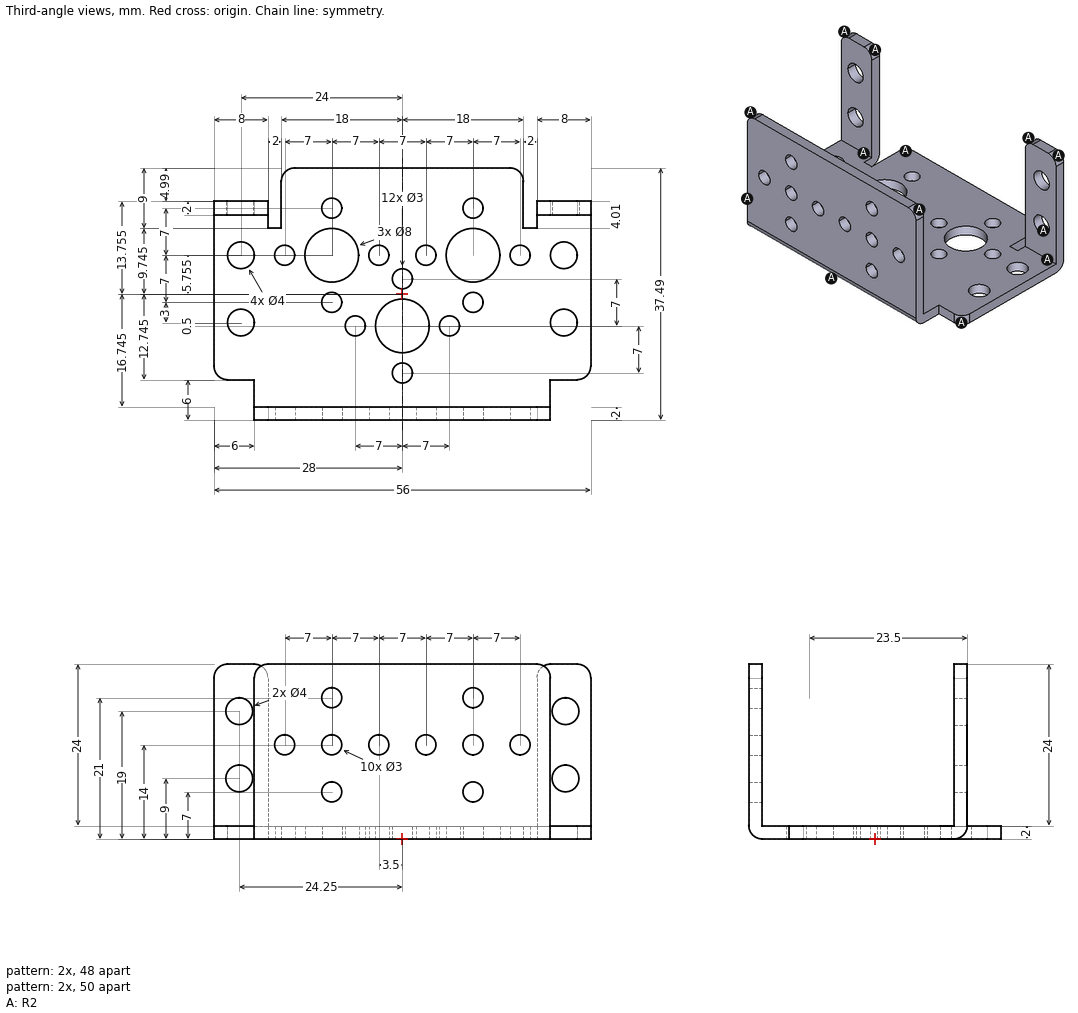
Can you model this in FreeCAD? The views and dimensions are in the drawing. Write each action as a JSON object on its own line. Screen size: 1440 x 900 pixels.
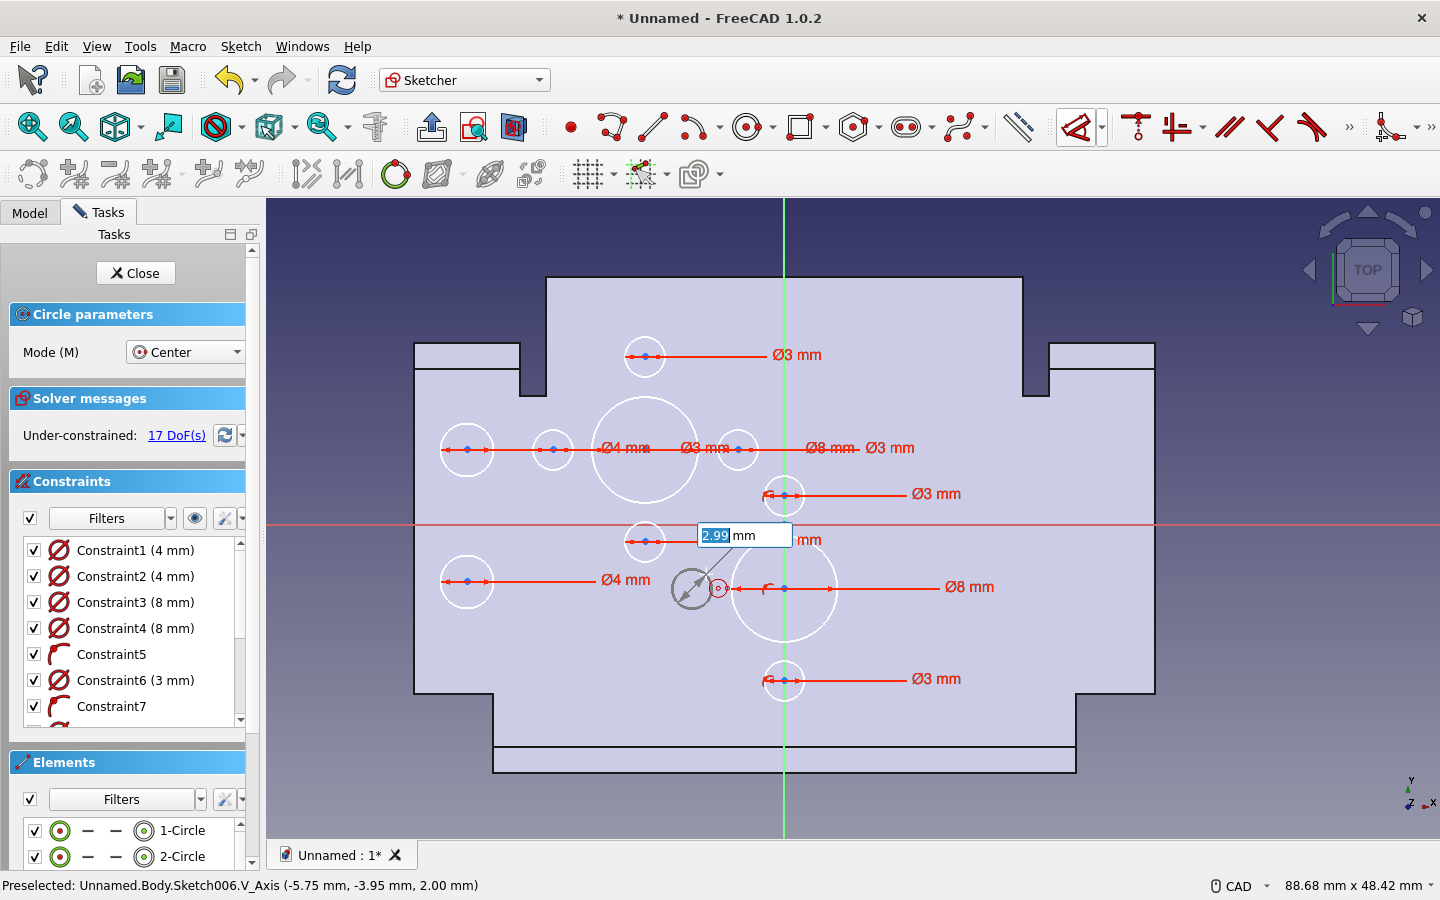
{"action": "type", "text": "3"}
{"action": "key", "text": "Return"}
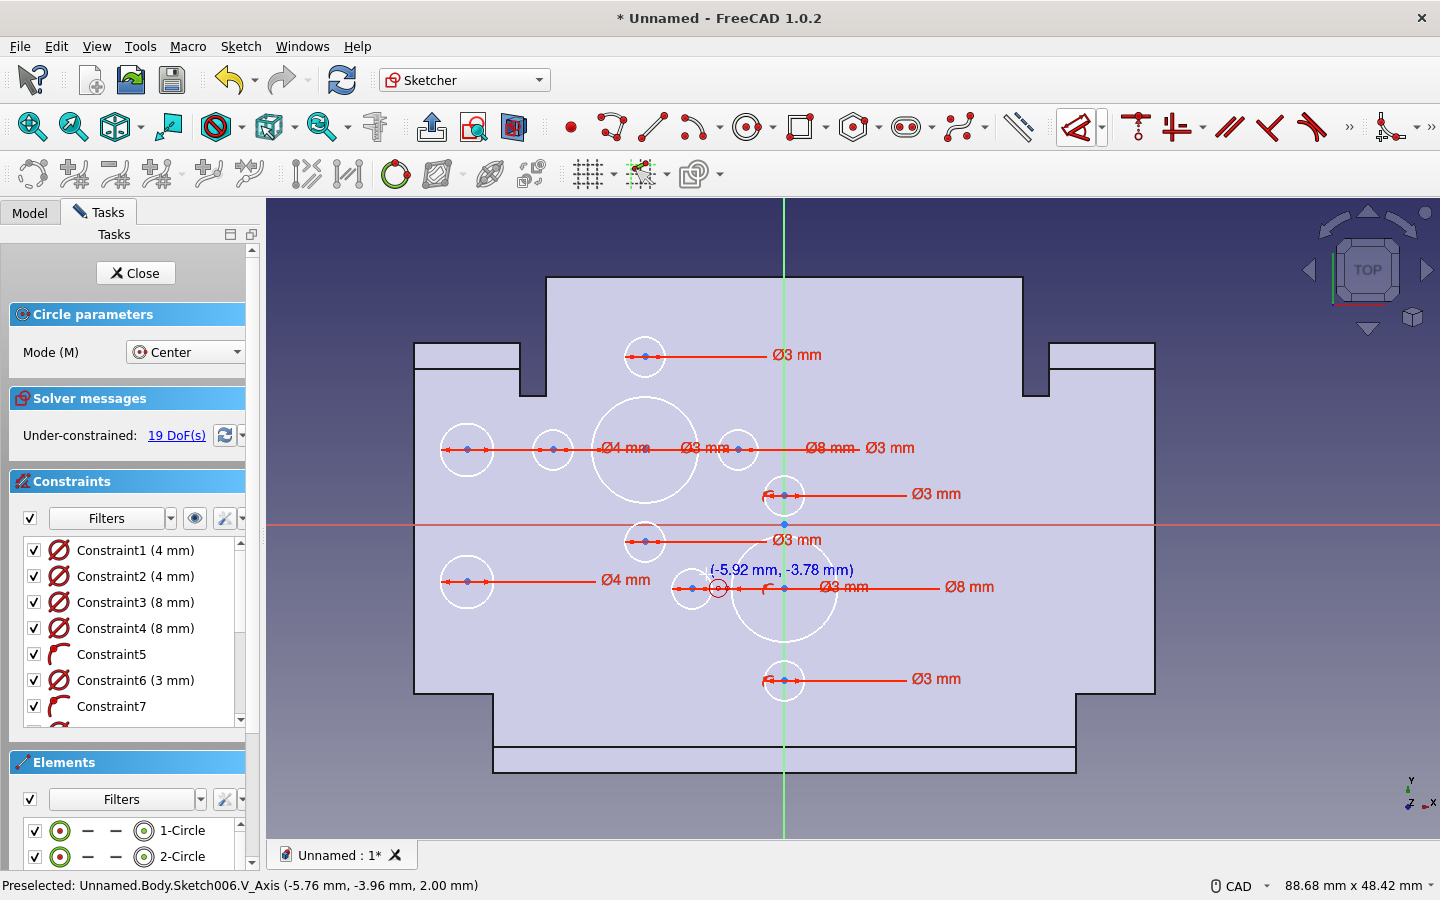
{"action": "left_click", "coordinate": [877, 588]}
{"action": "mouse_move", "coordinate": [891, 574]}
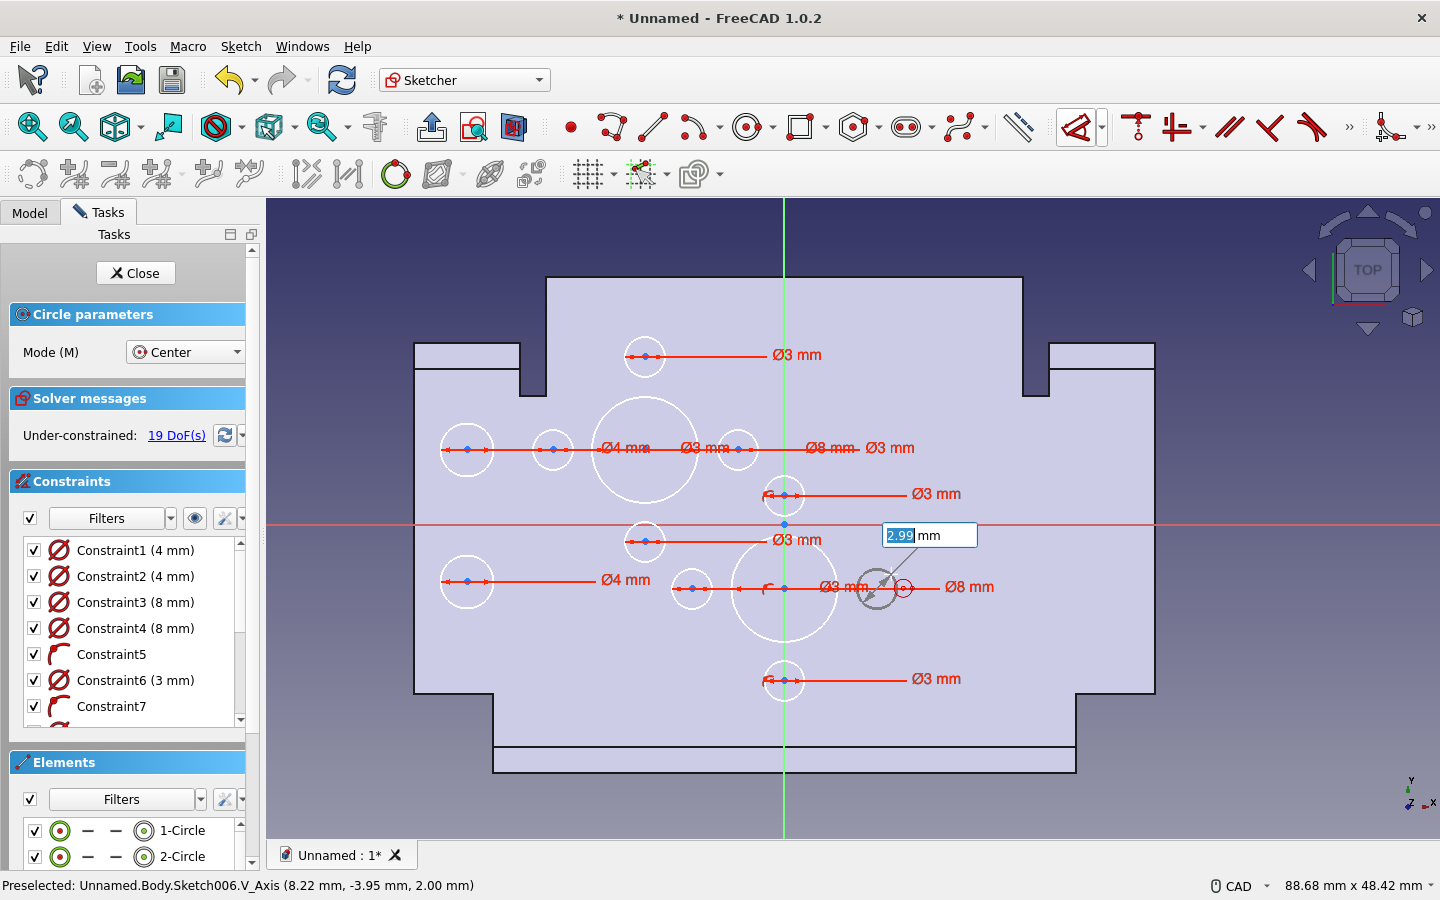
{"action": "type", "text": "3"}
{"action": "key", "text": "Return"}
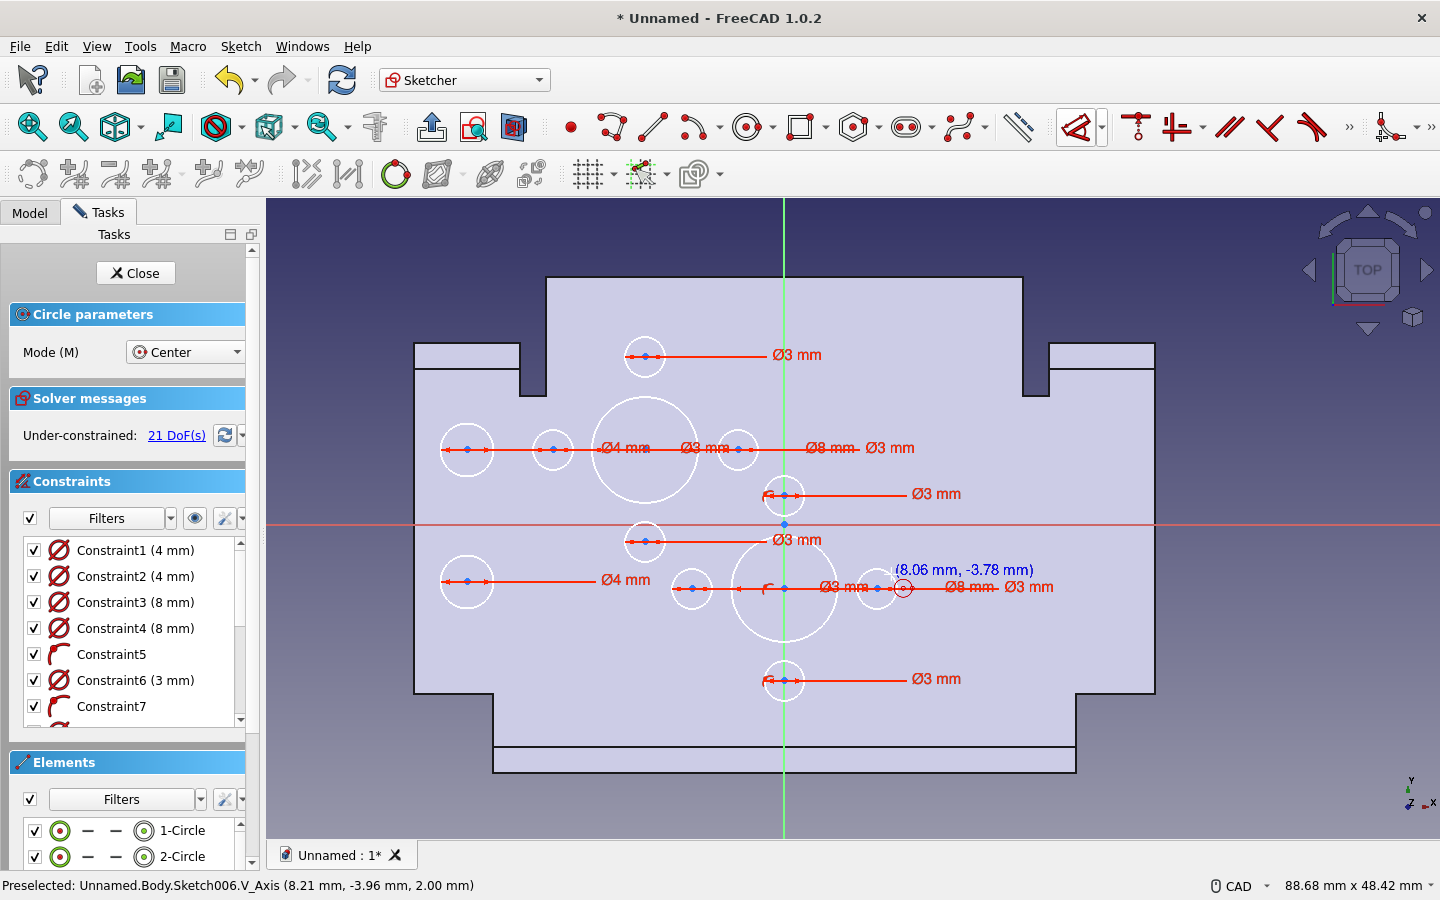
{"action": "left_click", "coordinate": [923, 356]}
{"action": "mouse_move", "coordinate": [937, 342]}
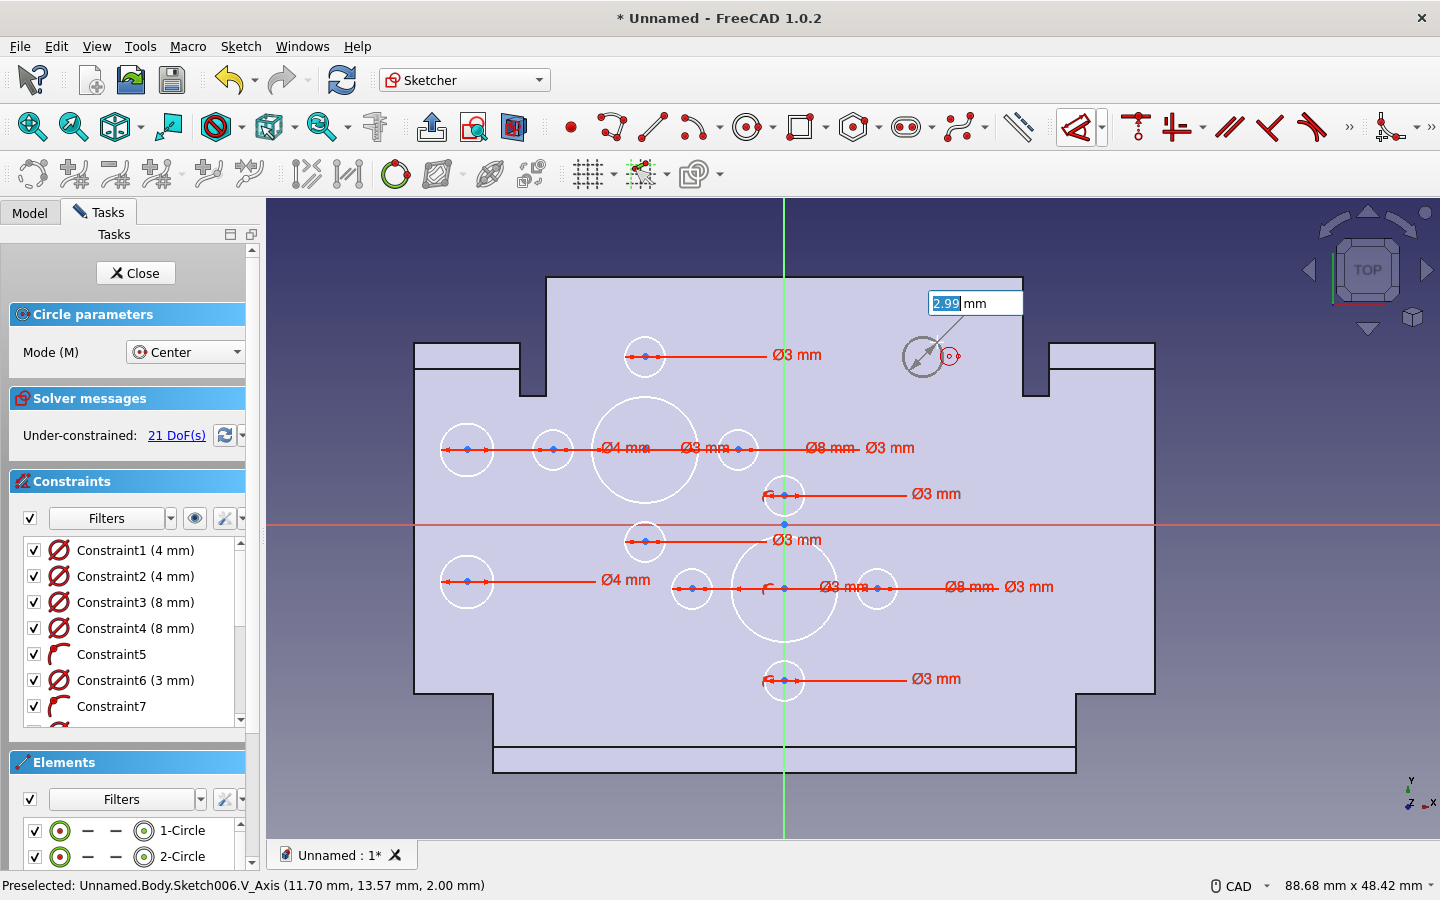
{"action": "type", "text": "3"}
{"action": "key", "text": "Return"}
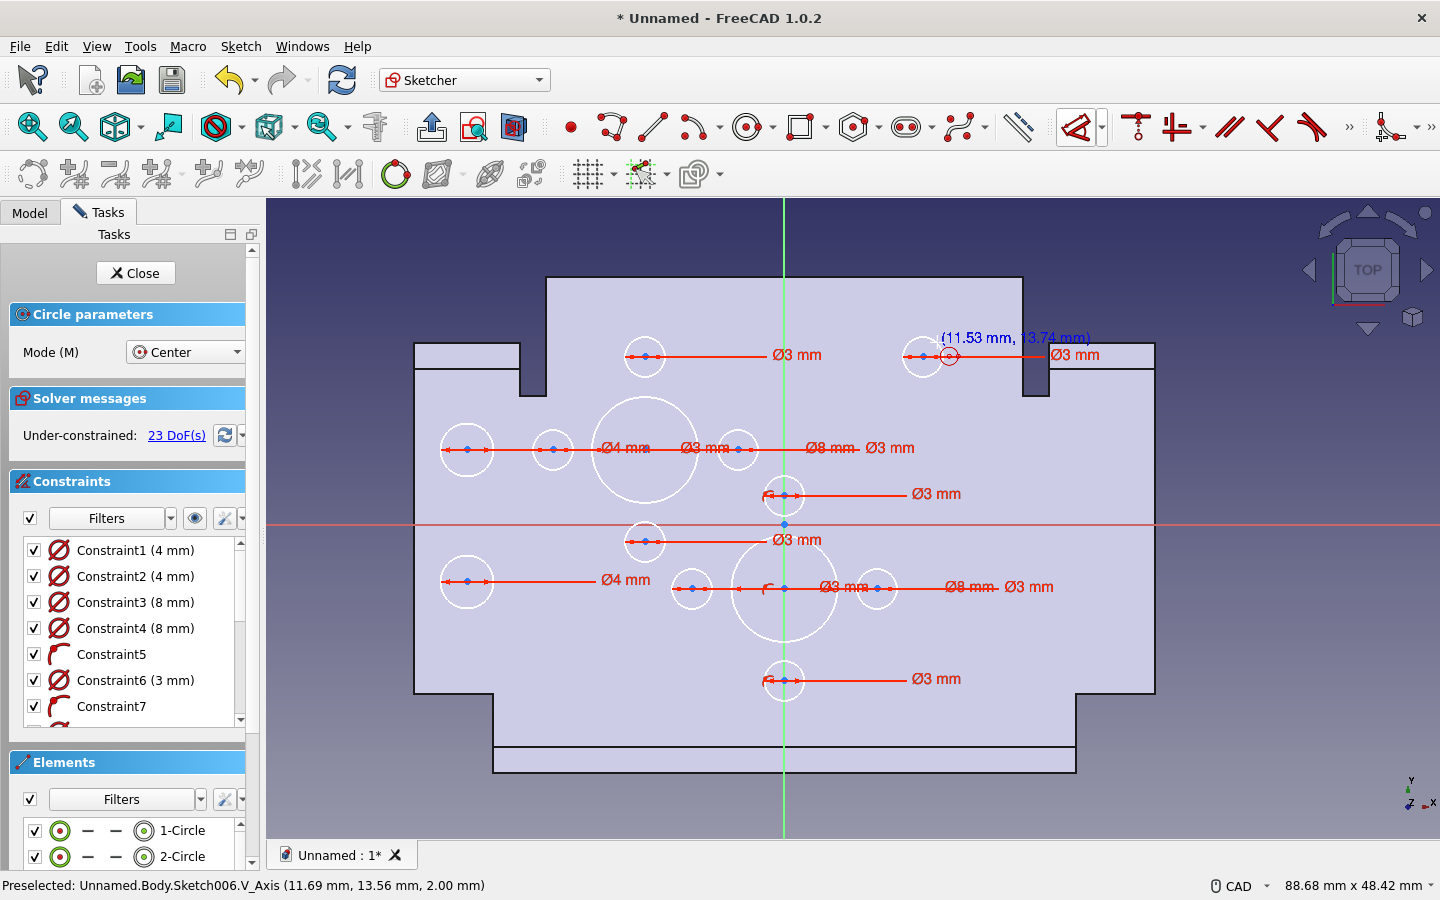
{"action": "left_click", "coordinate": [831, 449]}
{"action": "mouse_move", "coordinate": [845, 435]}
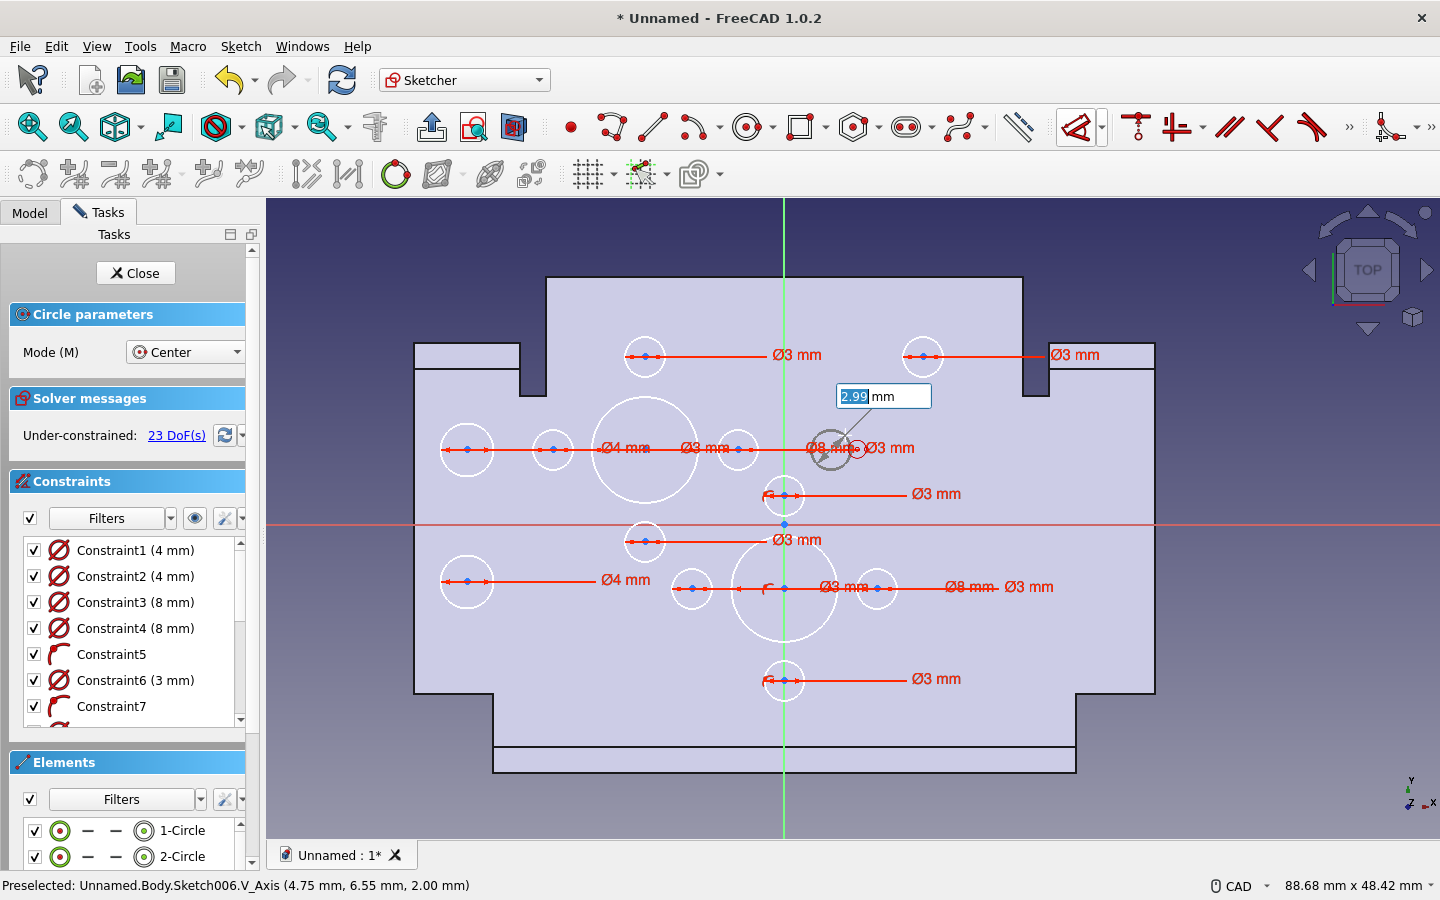
{"action": "type", "text": "3"}
{"action": "key", "text": "Return"}